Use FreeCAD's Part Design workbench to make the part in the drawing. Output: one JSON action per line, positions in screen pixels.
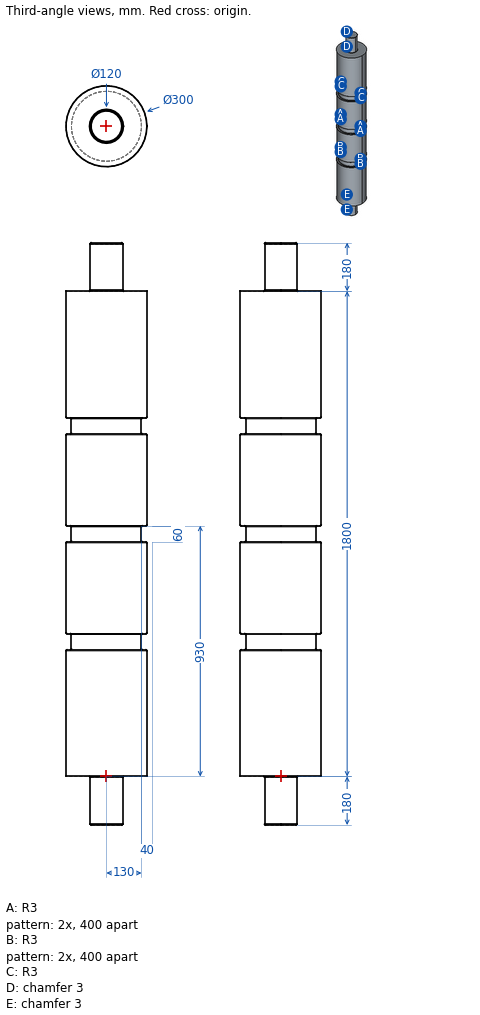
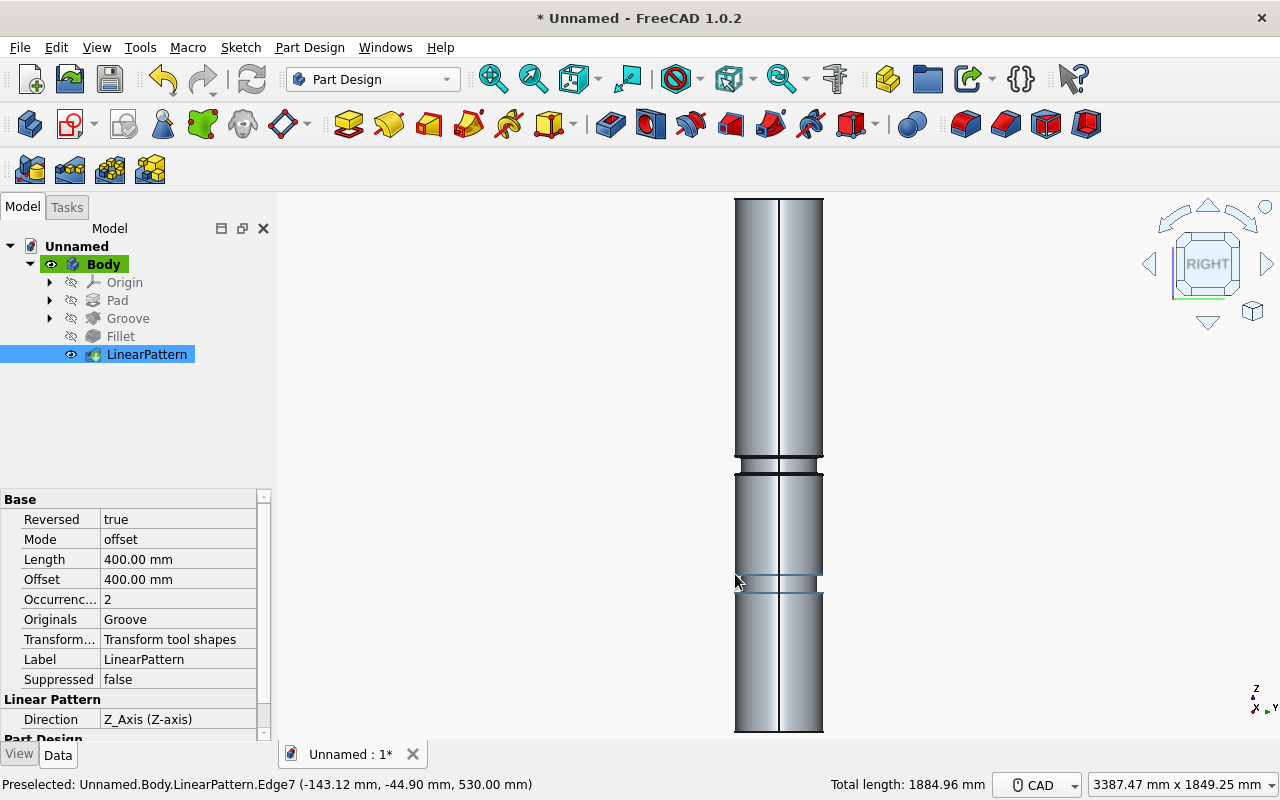
{"action": "key", "text": "5"}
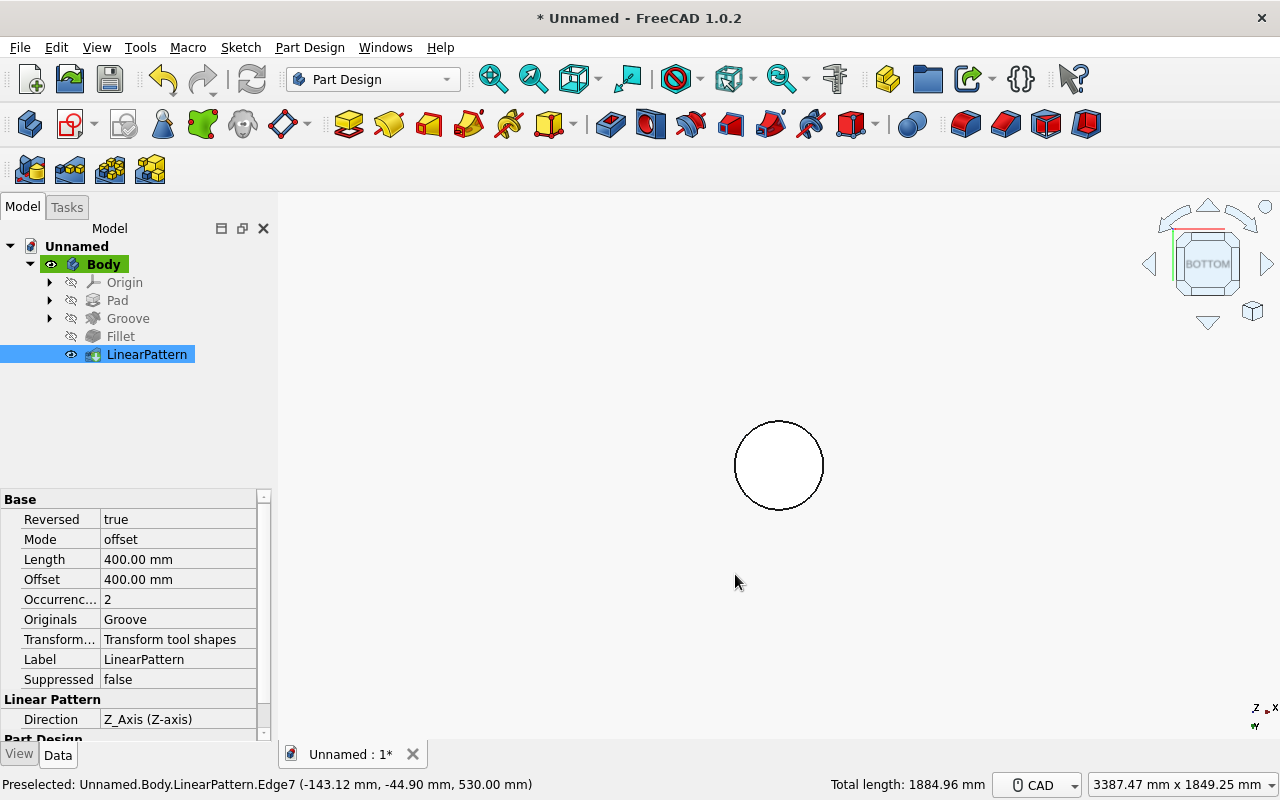
{"action": "left_click", "coordinate": [494, 80]}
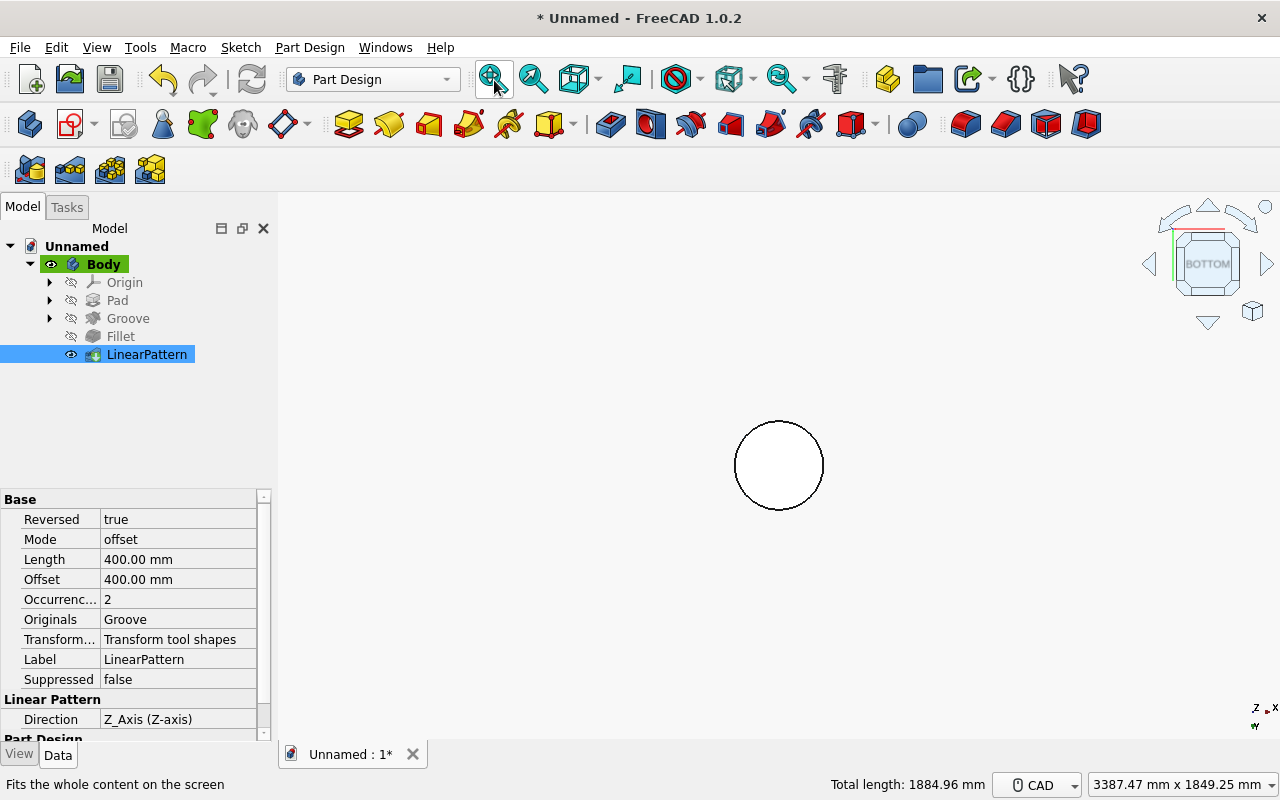
{"action": "key", "text": "4"}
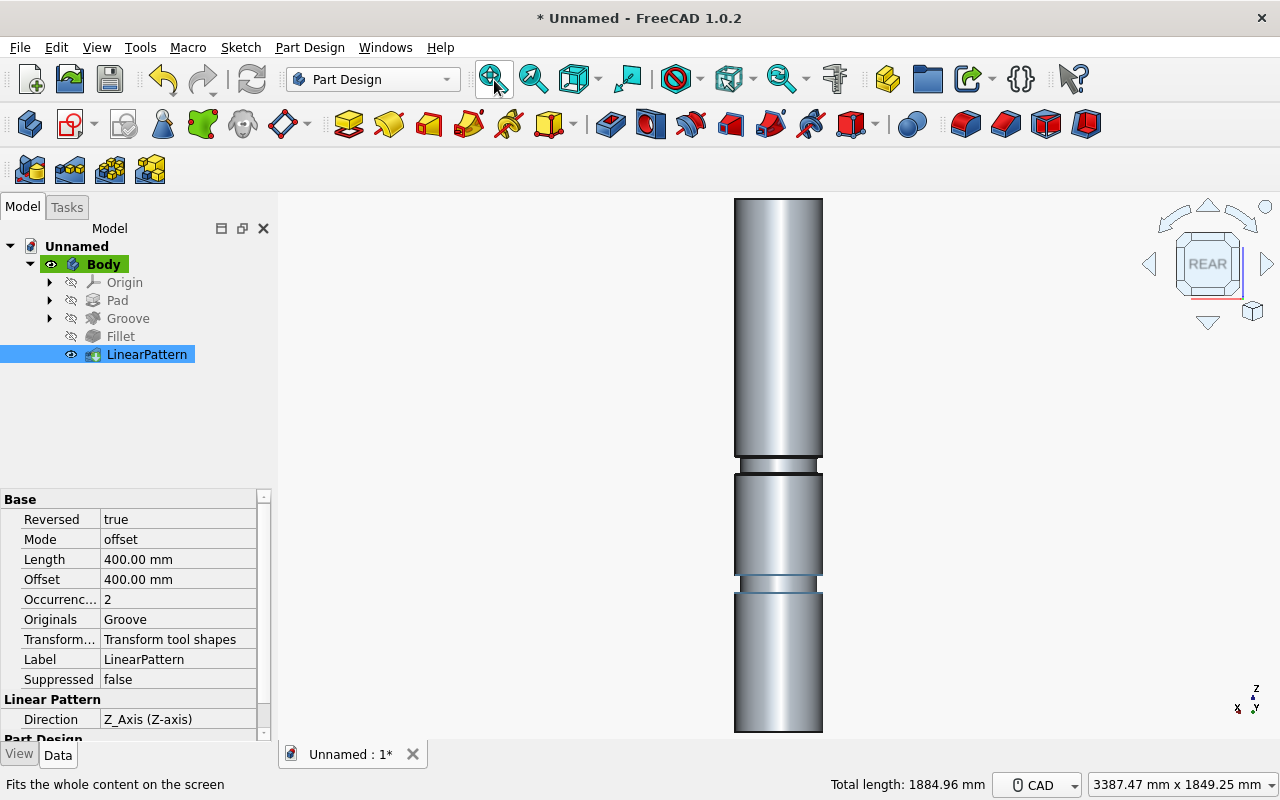
{"action": "key", "text": "6"}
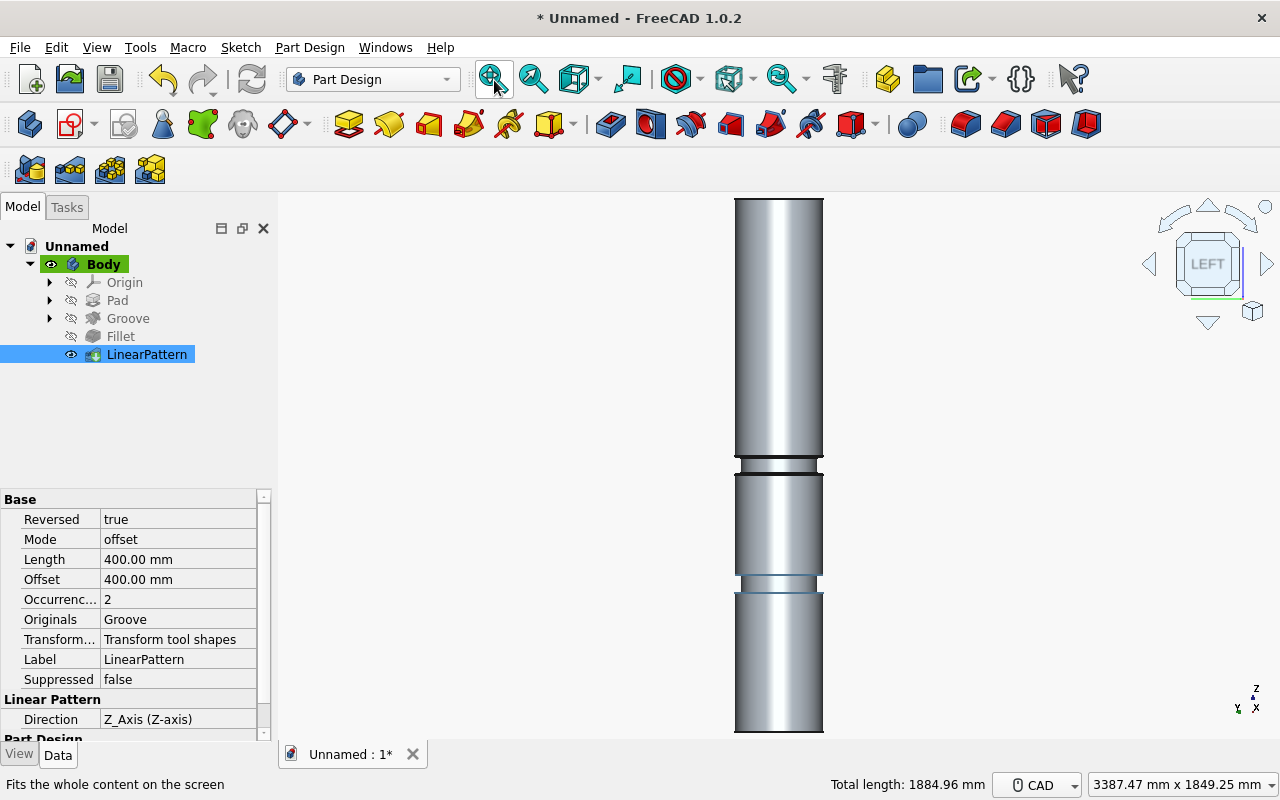
{"action": "key", "text": "v 3"}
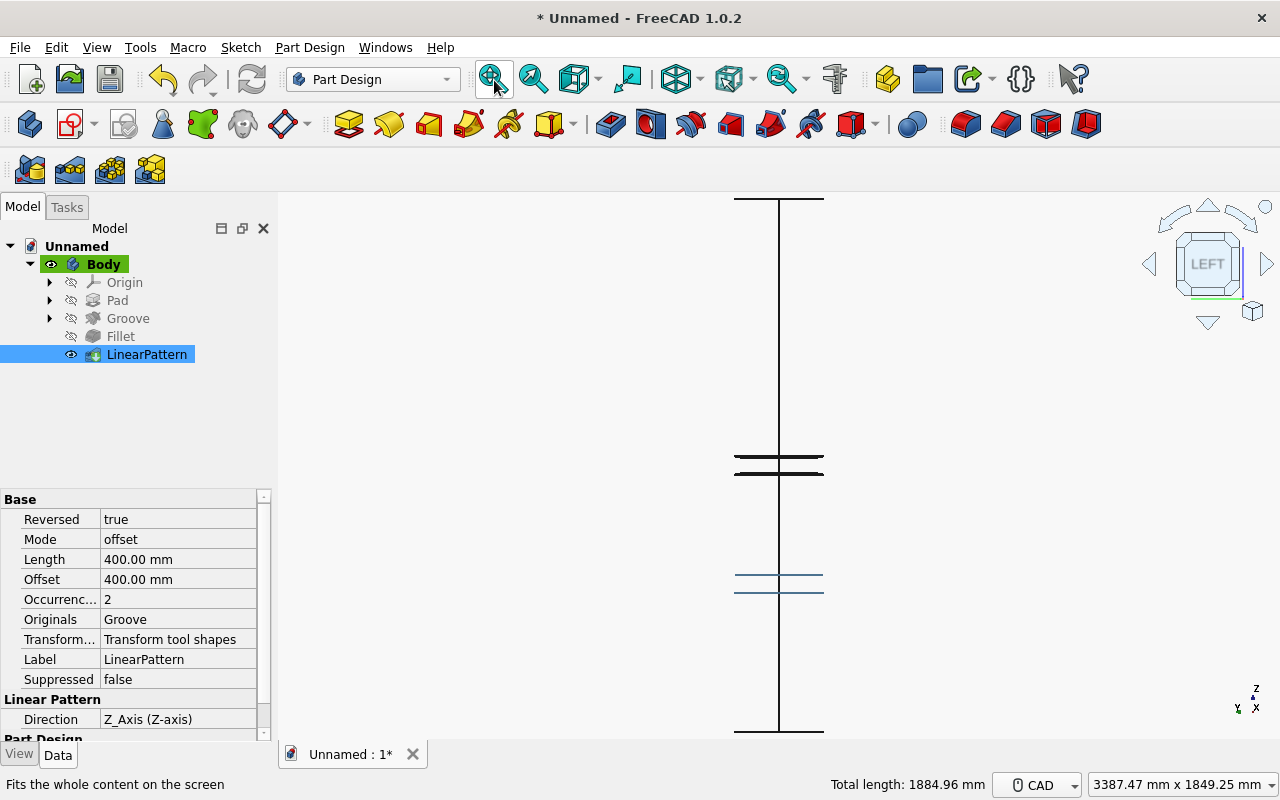
{"action": "key", "text": "0"}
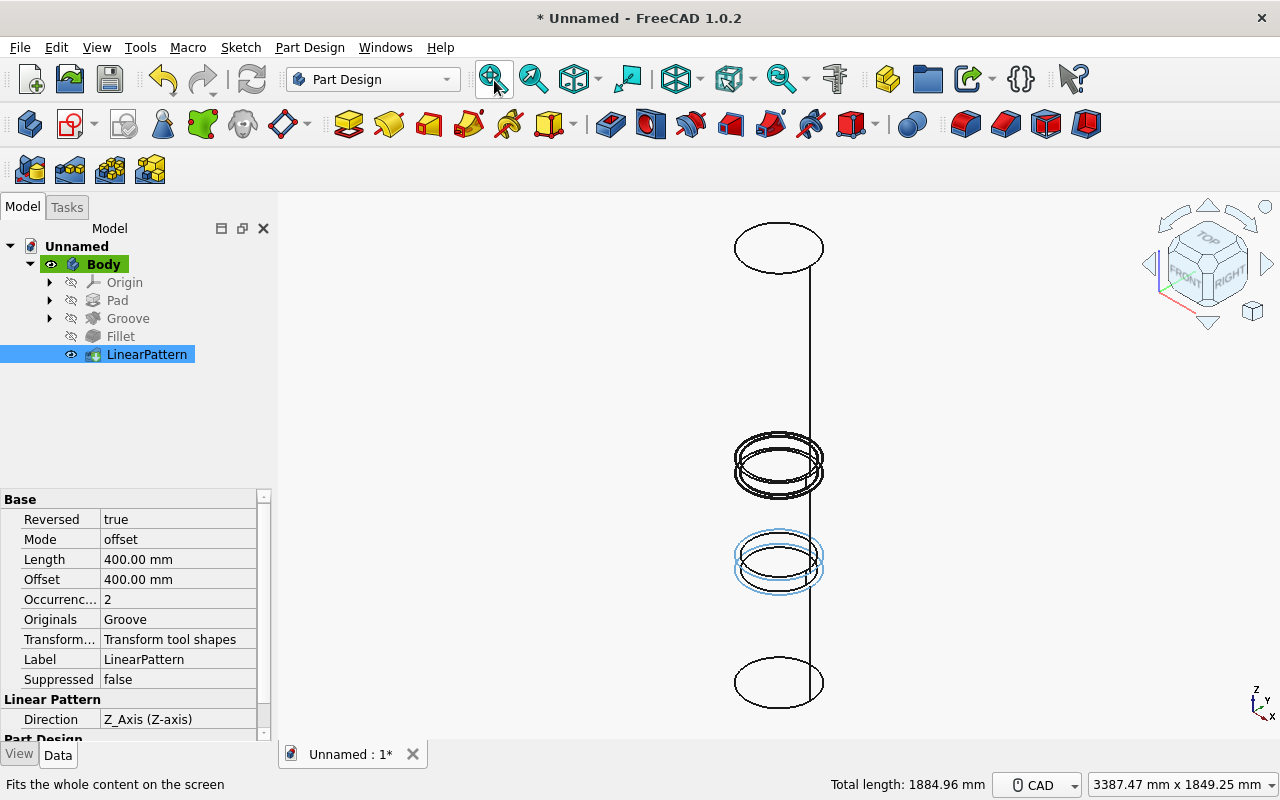
{"action": "left_click", "coordinate": [752, 538], "text": "ctrl"}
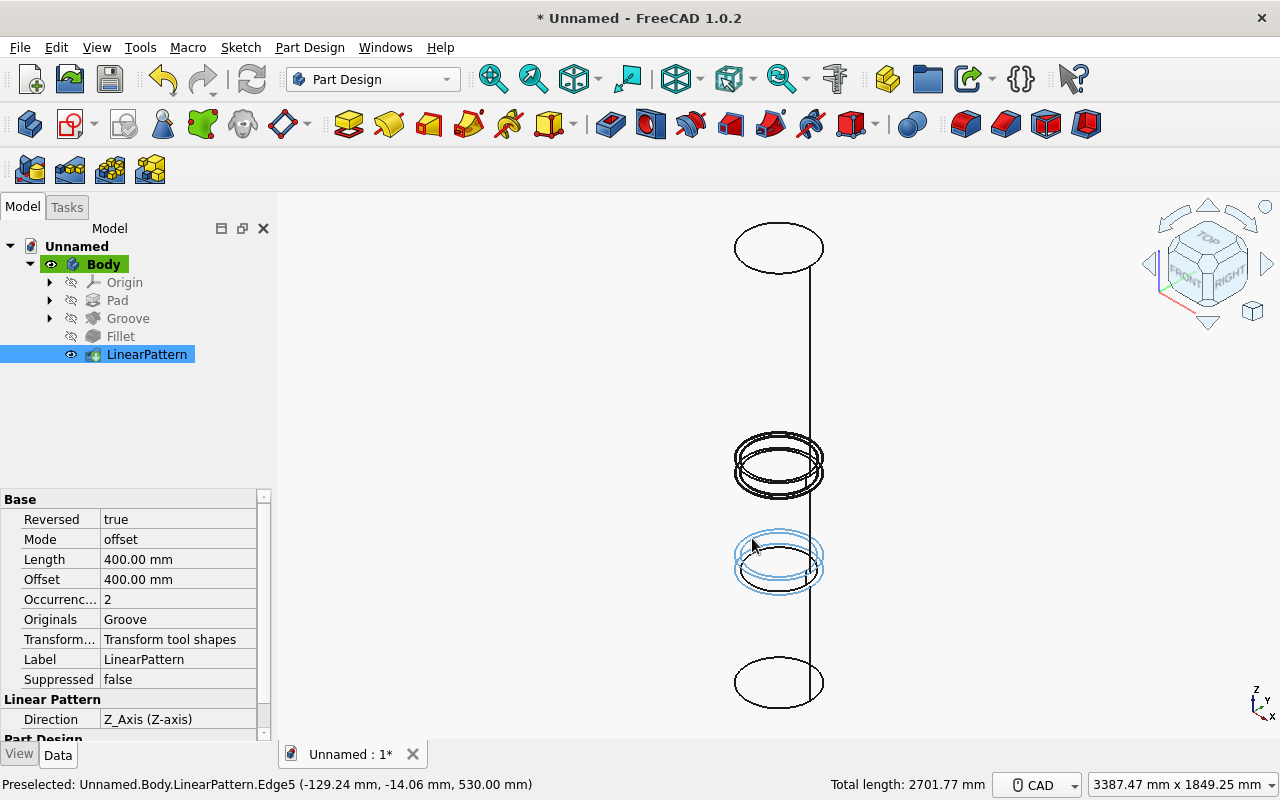
{"action": "left_click", "coordinate": [752, 553], "text": "ctrl"}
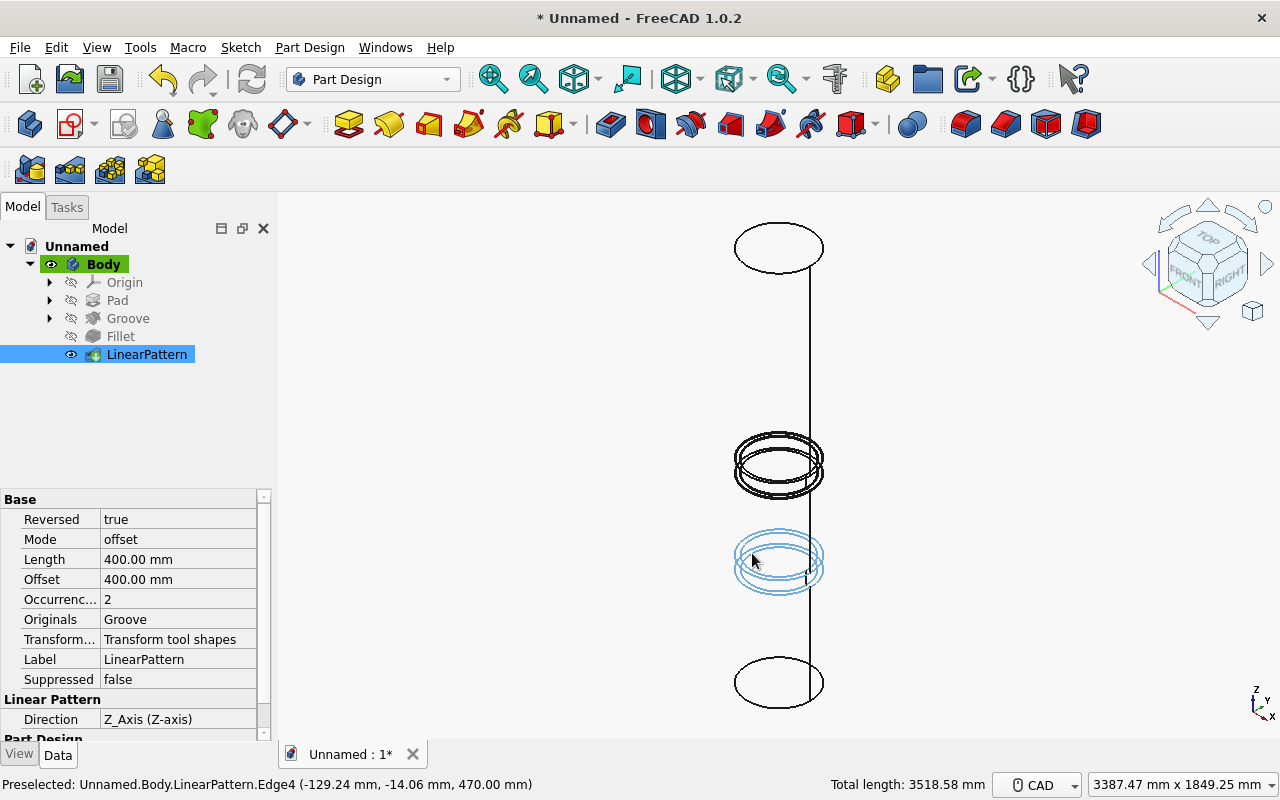
{"action": "key", "text": "v 1"}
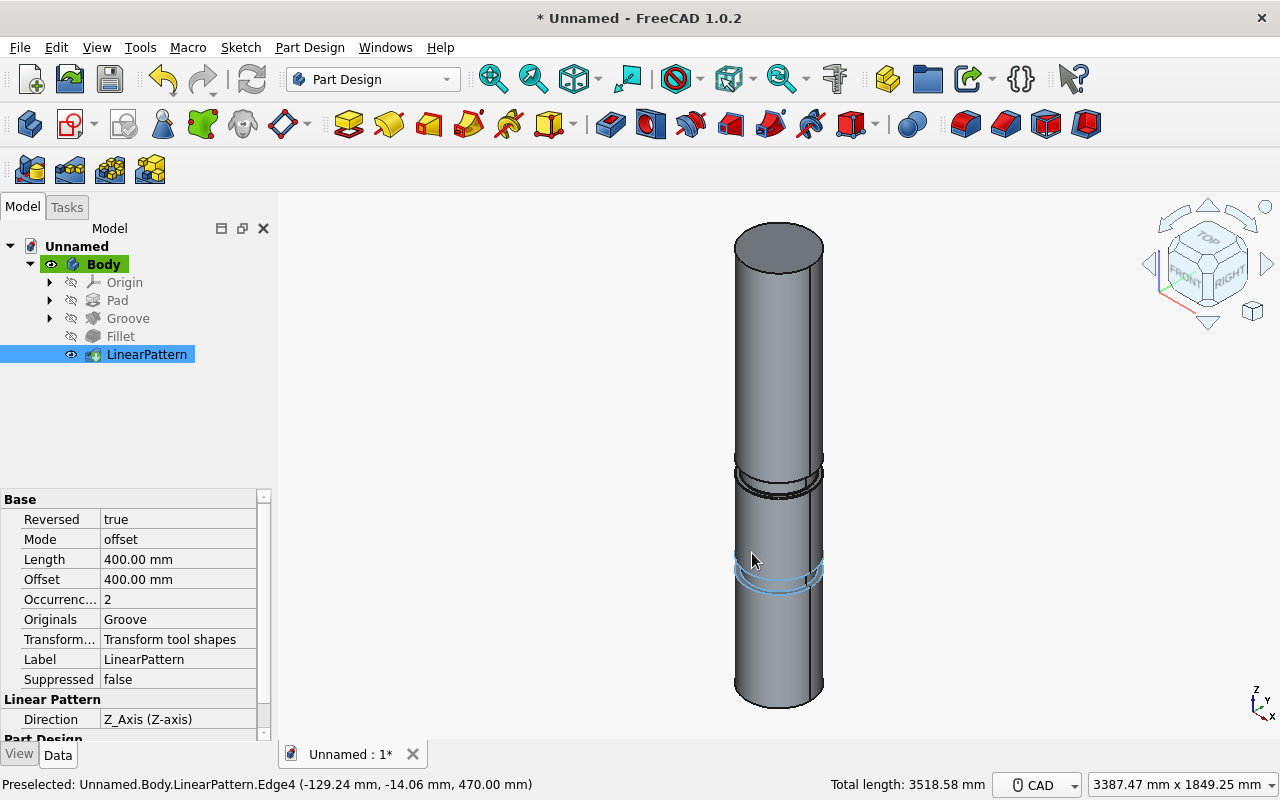
{"action": "left_click", "coordinate": [966, 124]}